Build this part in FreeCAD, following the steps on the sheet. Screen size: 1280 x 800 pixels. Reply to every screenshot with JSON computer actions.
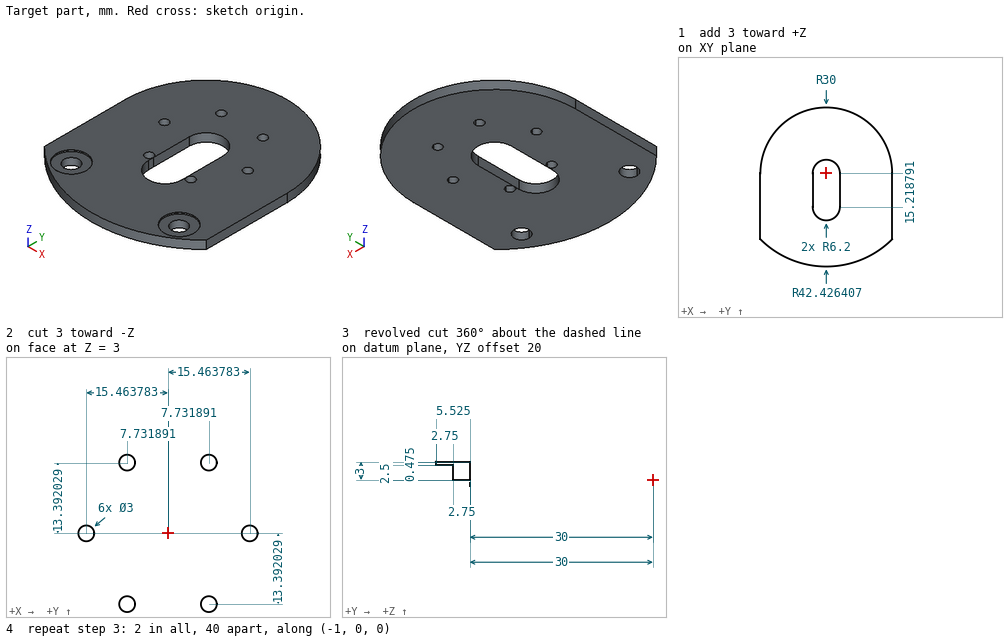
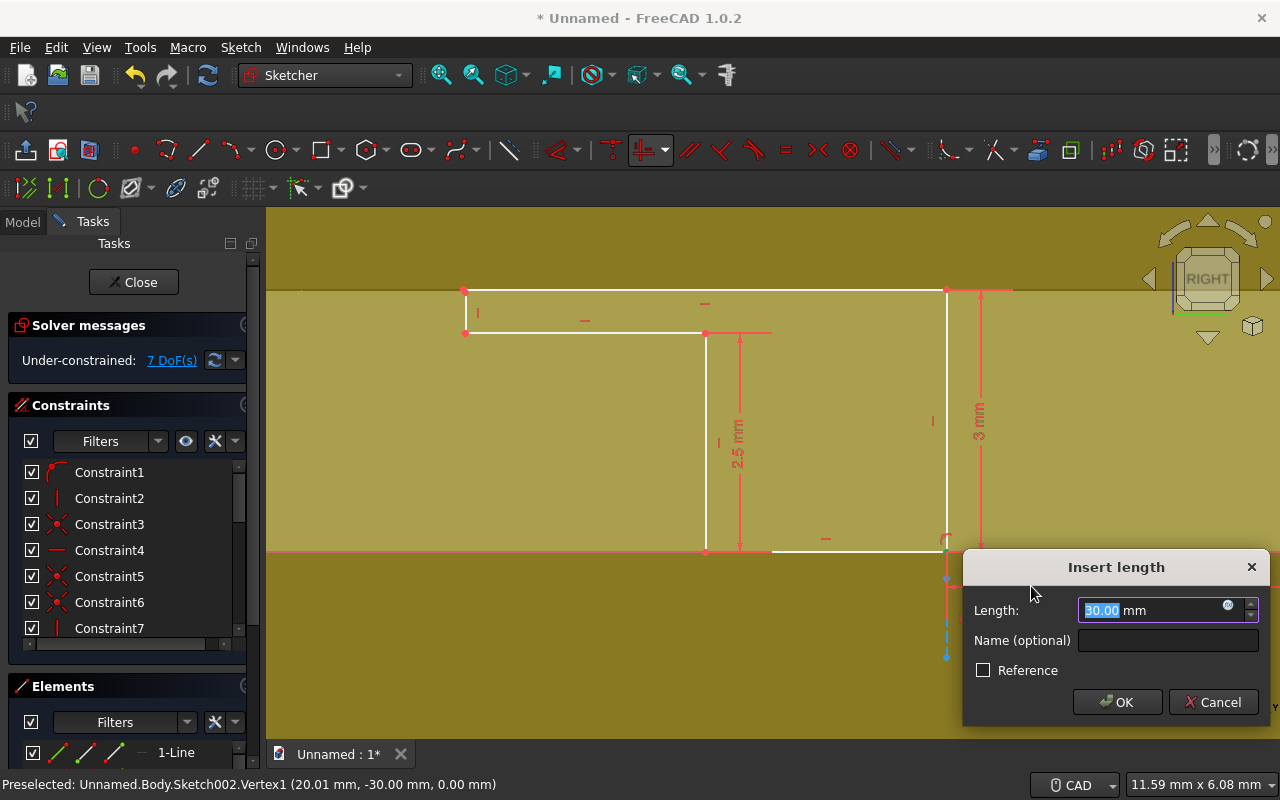
{"action": "type", "text": "30"}
{"action": "key", "text": "Return"}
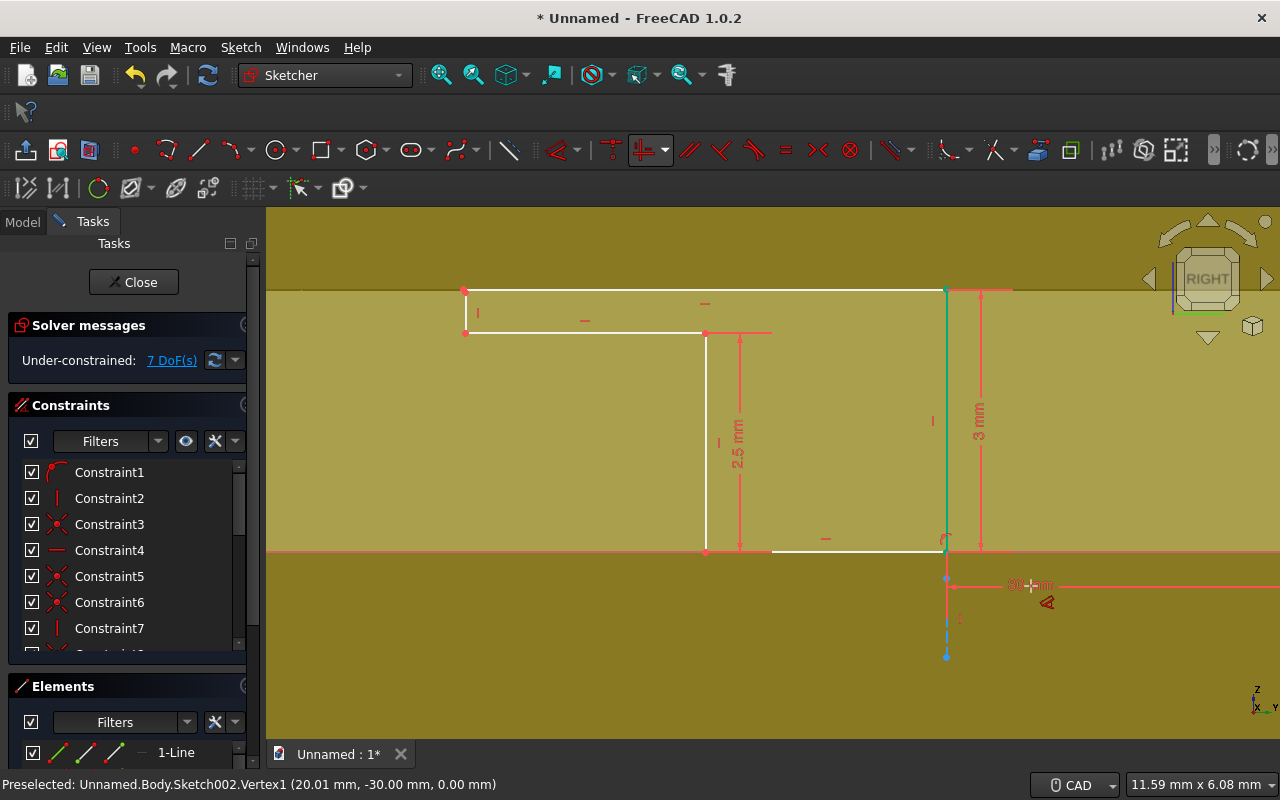
{"action": "left_click", "coordinate": [947, 579]}
{"action": "left_click", "coordinate": [1031, 613]}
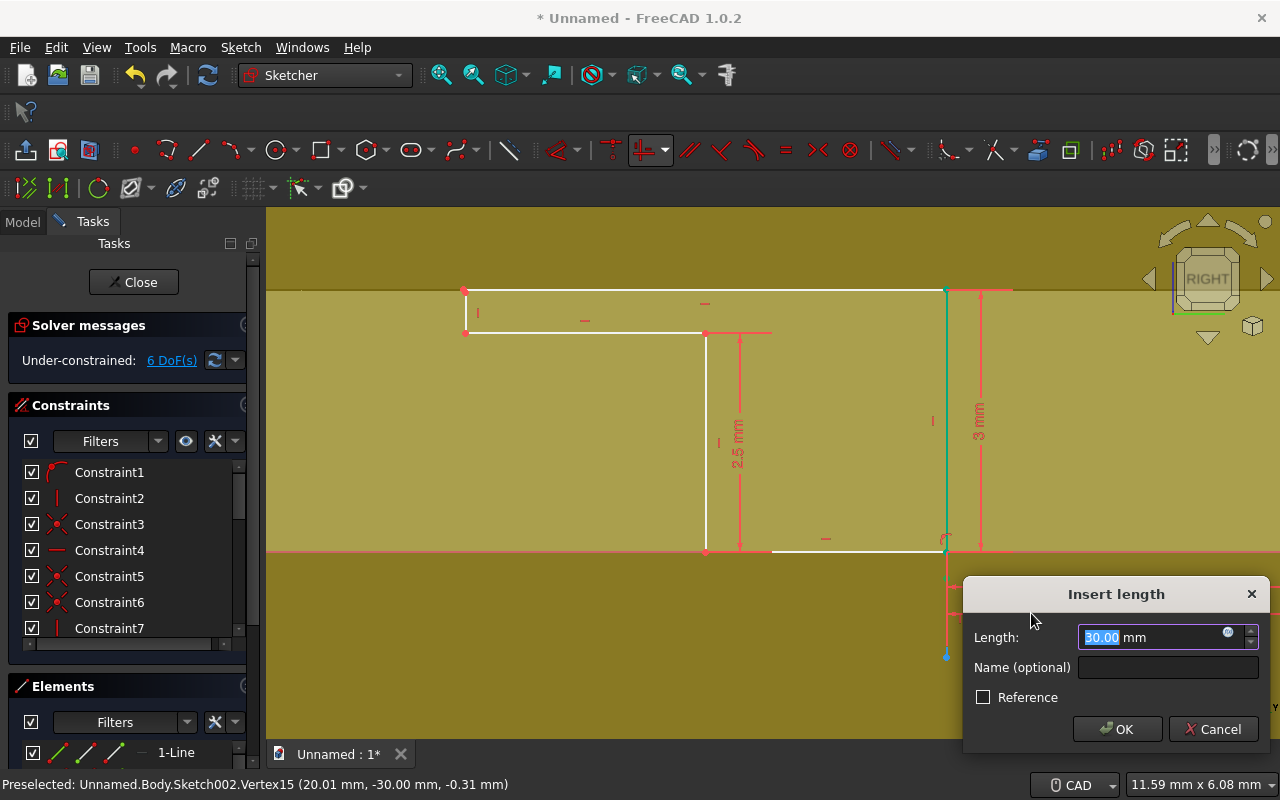
{"action": "type", "text": "30"}
{"action": "key", "text": "Return"}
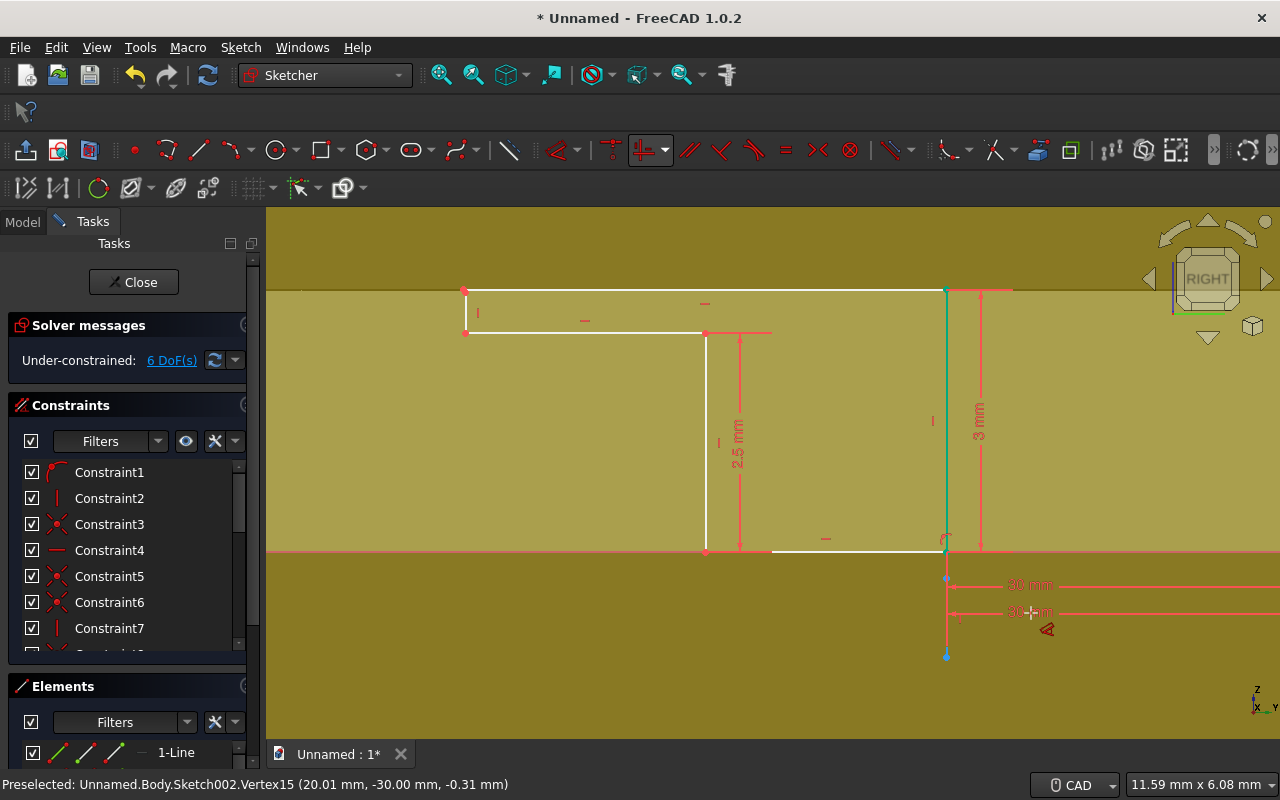
{"action": "left_click", "coordinate": [538, 333]}
{"action": "left_click", "coordinate": [586, 367]}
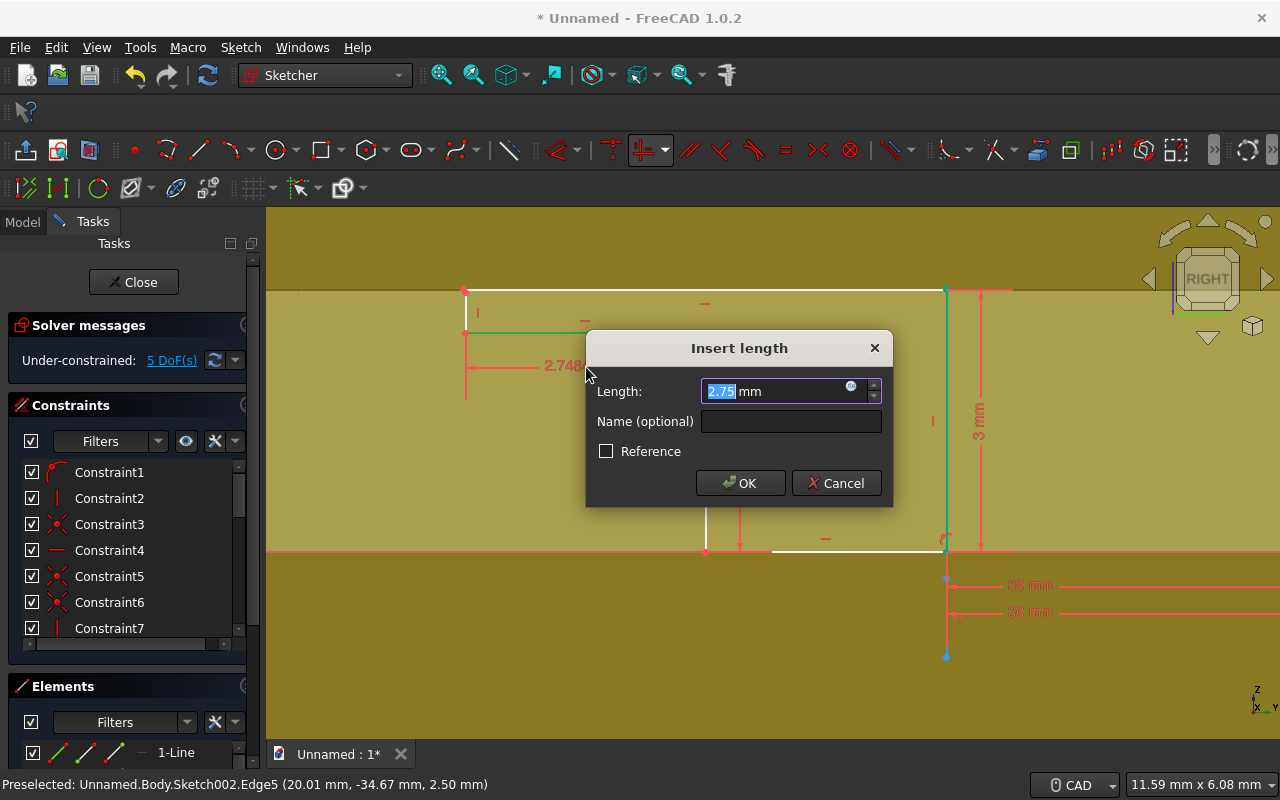
{"action": "type", "text": "2.75"}
{"action": "key", "text": "Return"}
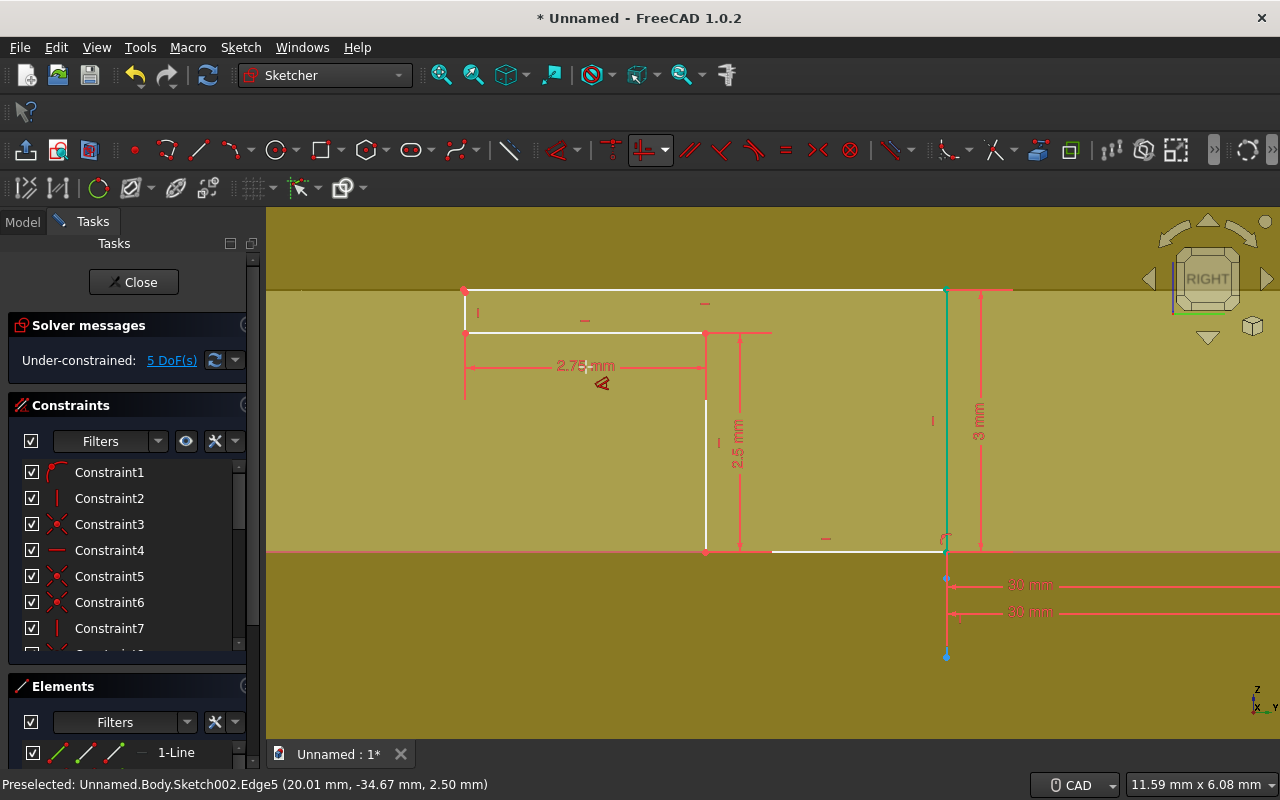
{"action": "left_click", "coordinate": [778, 552]}
{"action": "left_click", "coordinate": [826, 586]}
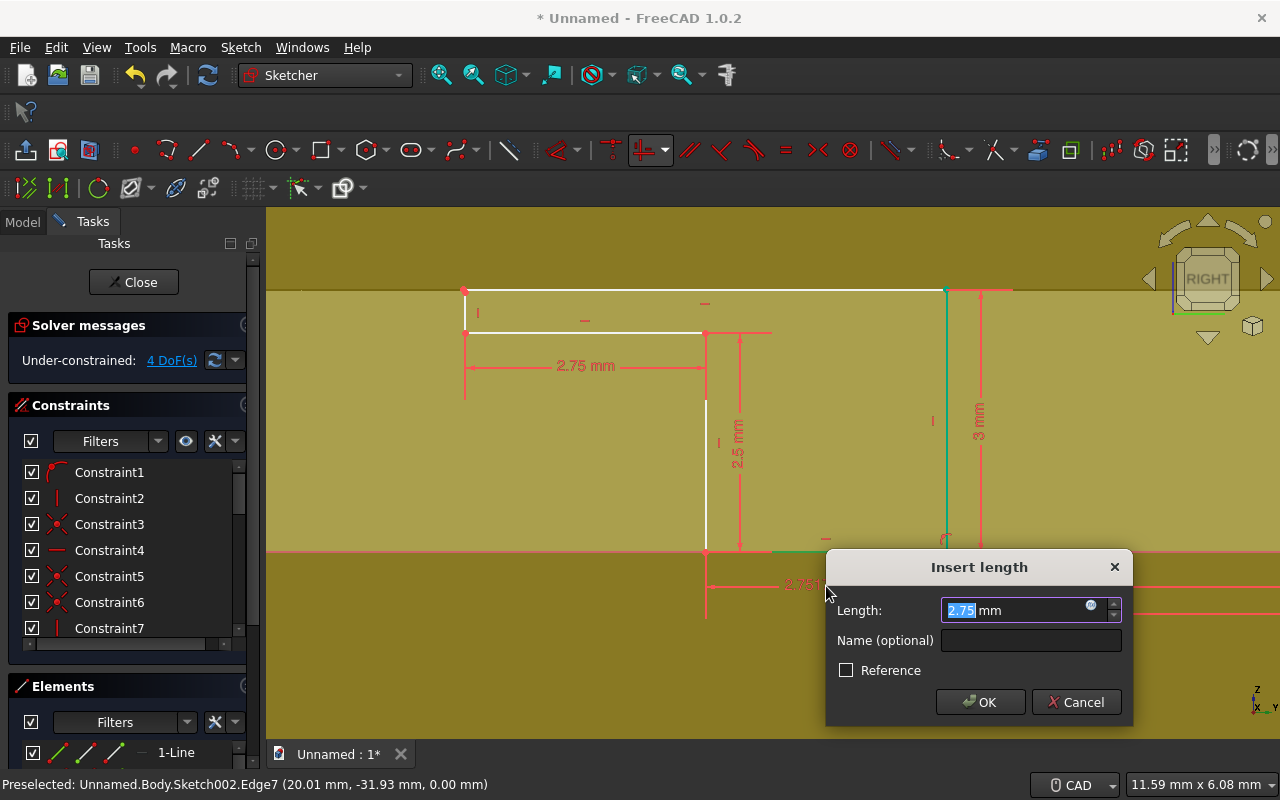
{"action": "type", "text": "2.75"}
{"action": "key", "text": "Return"}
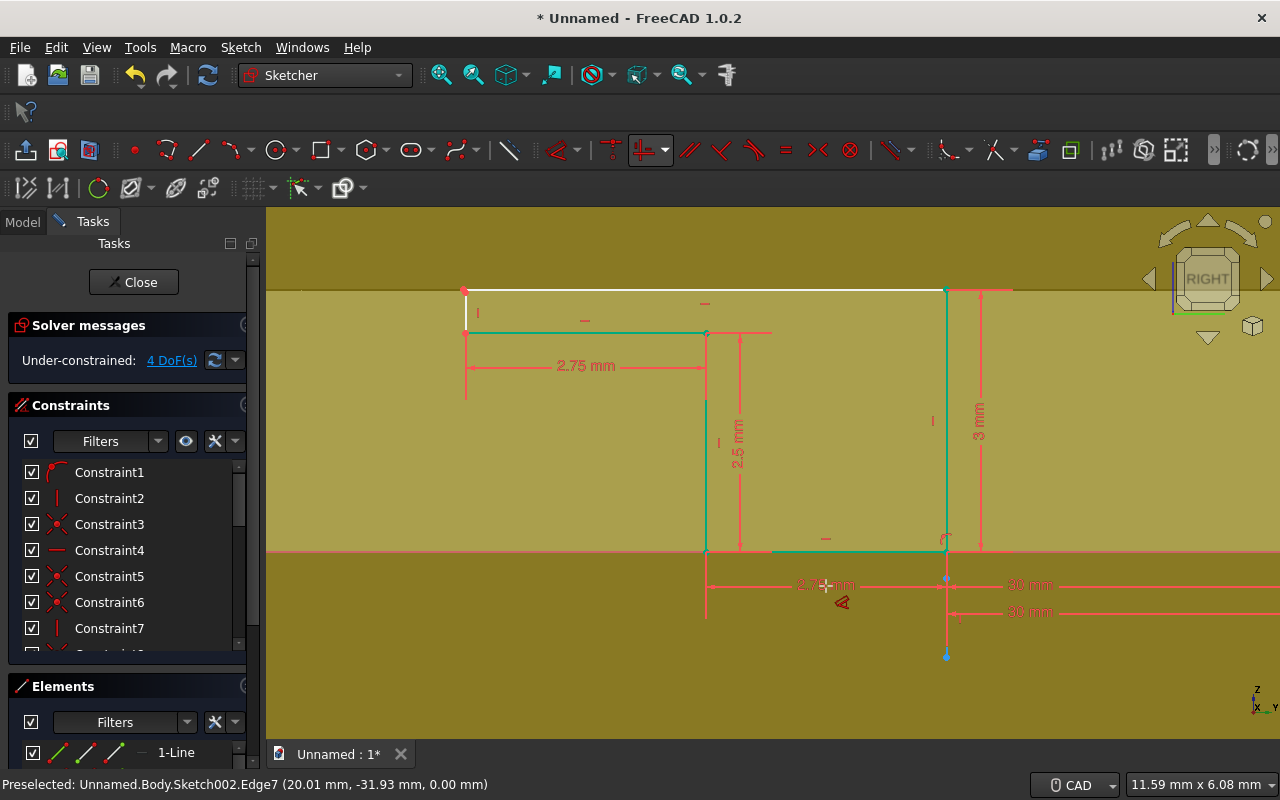
{"action": "left_click", "coordinate": [802, 290]}
{"action": "left_click", "coordinate": [705, 256]}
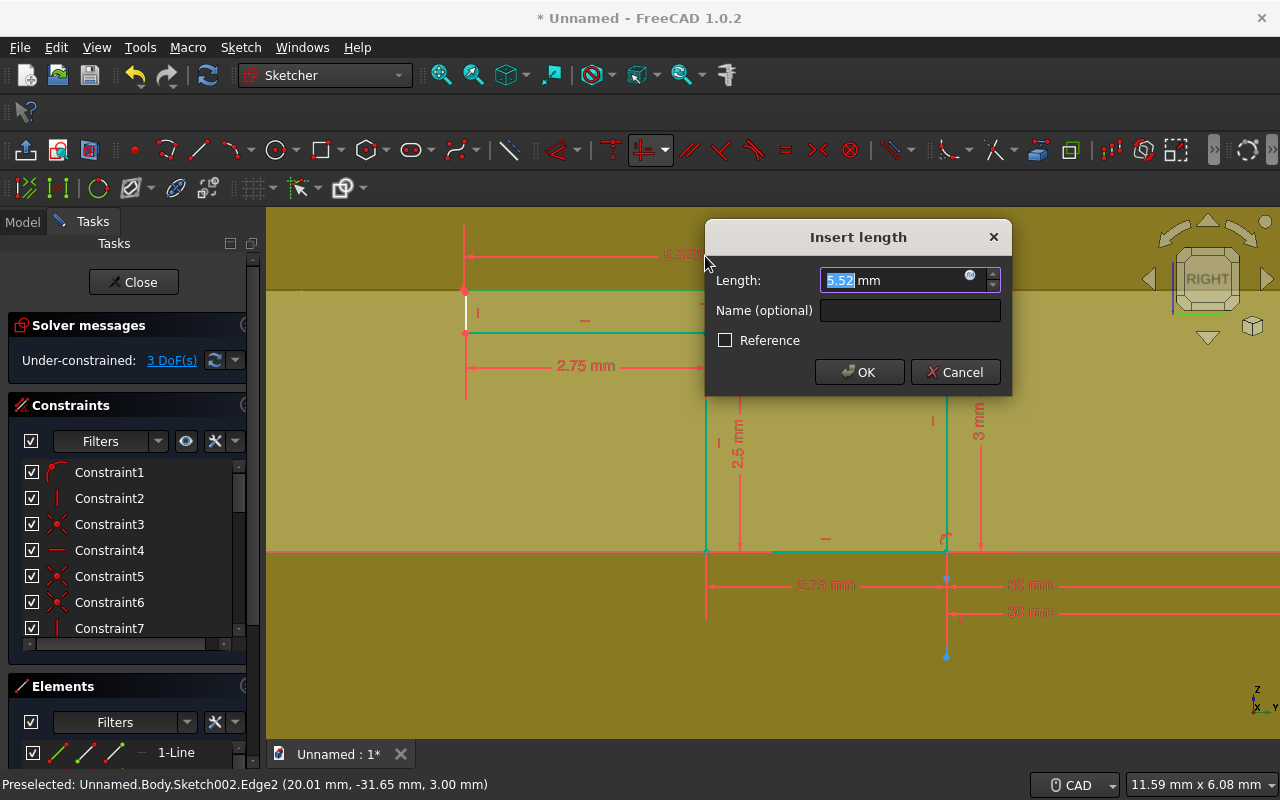
{"action": "type", "text": "5.525"}
{"action": "key", "text": "Return"}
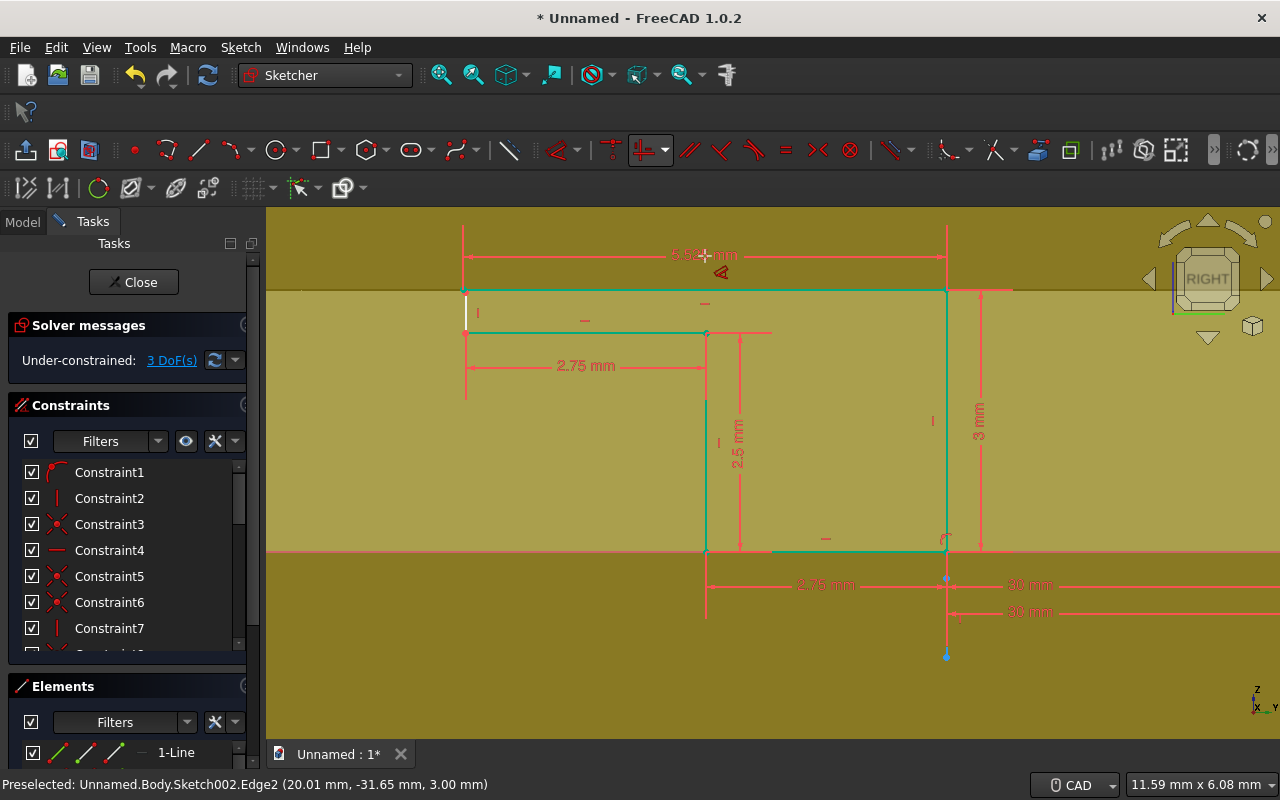
{"action": "left_click", "coordinate": [466, 304]}
{"action": "left_click", "coordinate": [432, 313]}